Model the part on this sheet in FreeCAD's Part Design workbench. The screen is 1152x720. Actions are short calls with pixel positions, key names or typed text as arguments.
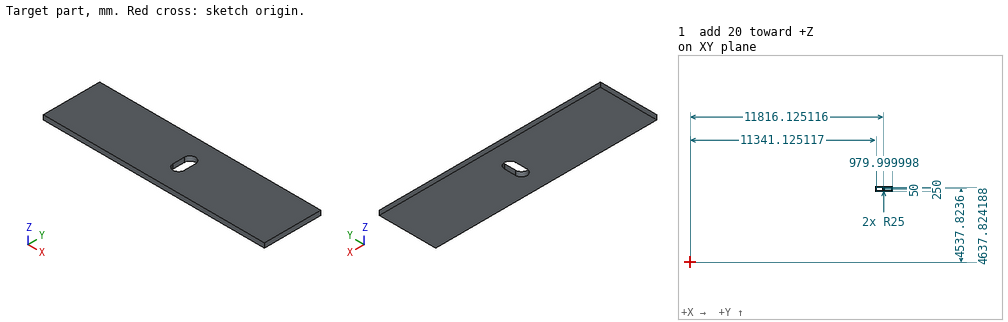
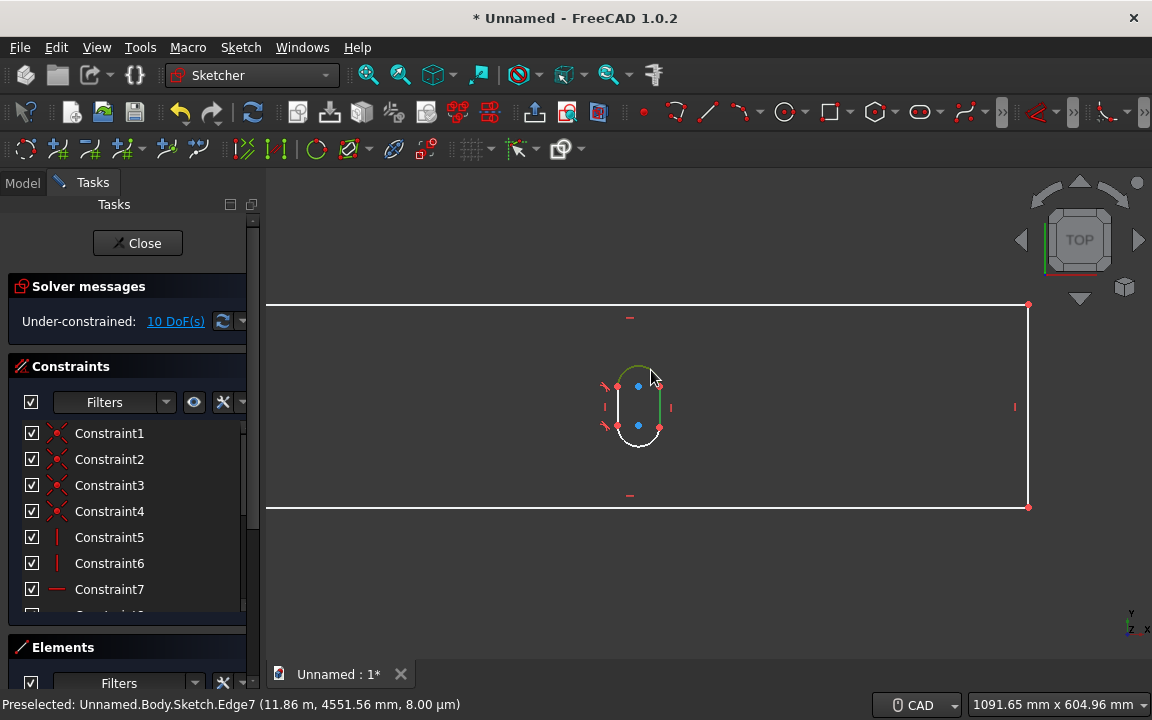
key(t)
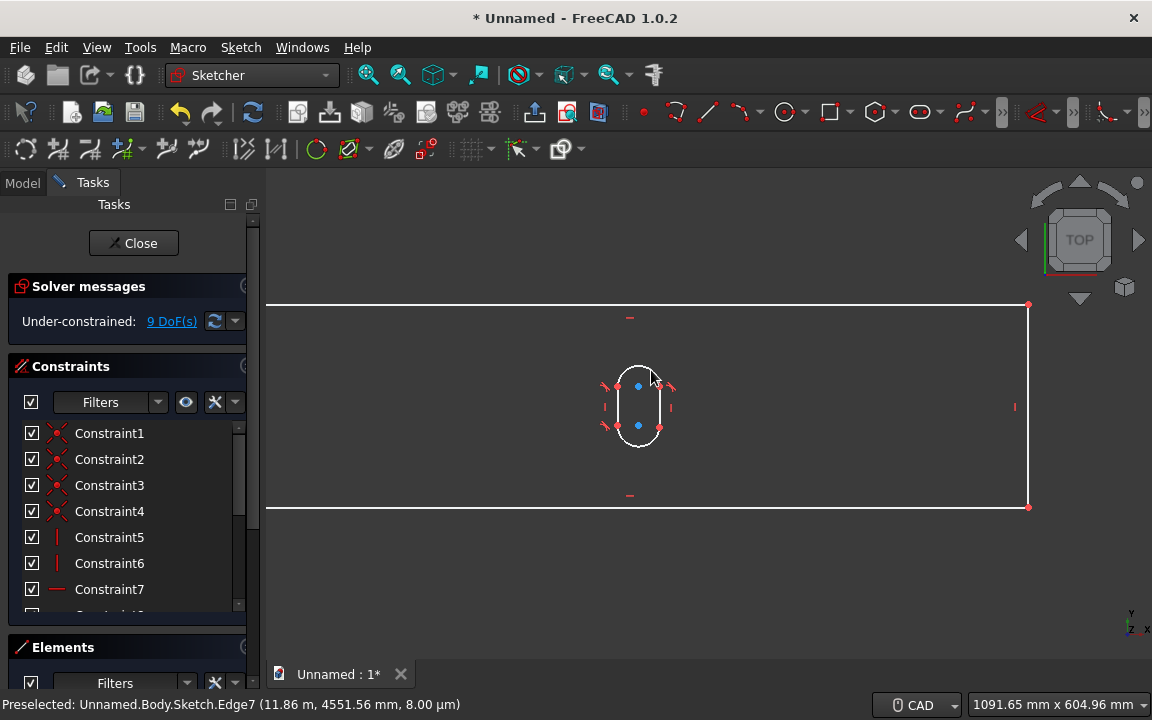
click(660, 399)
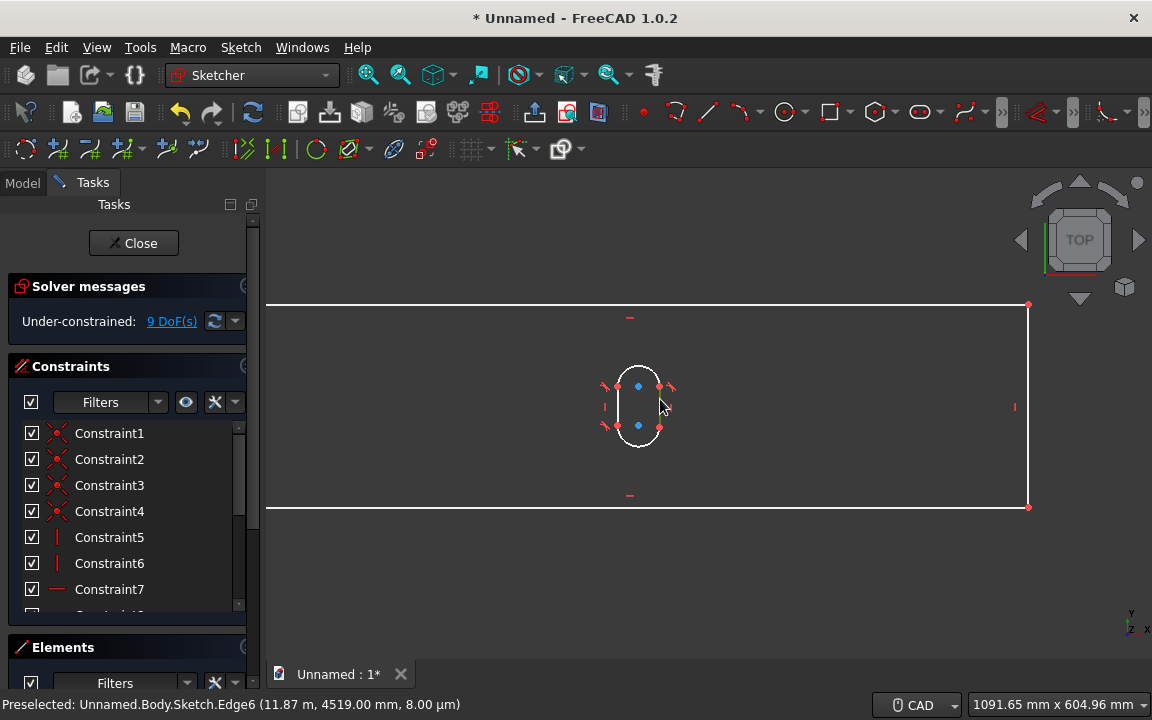
click(626, 442)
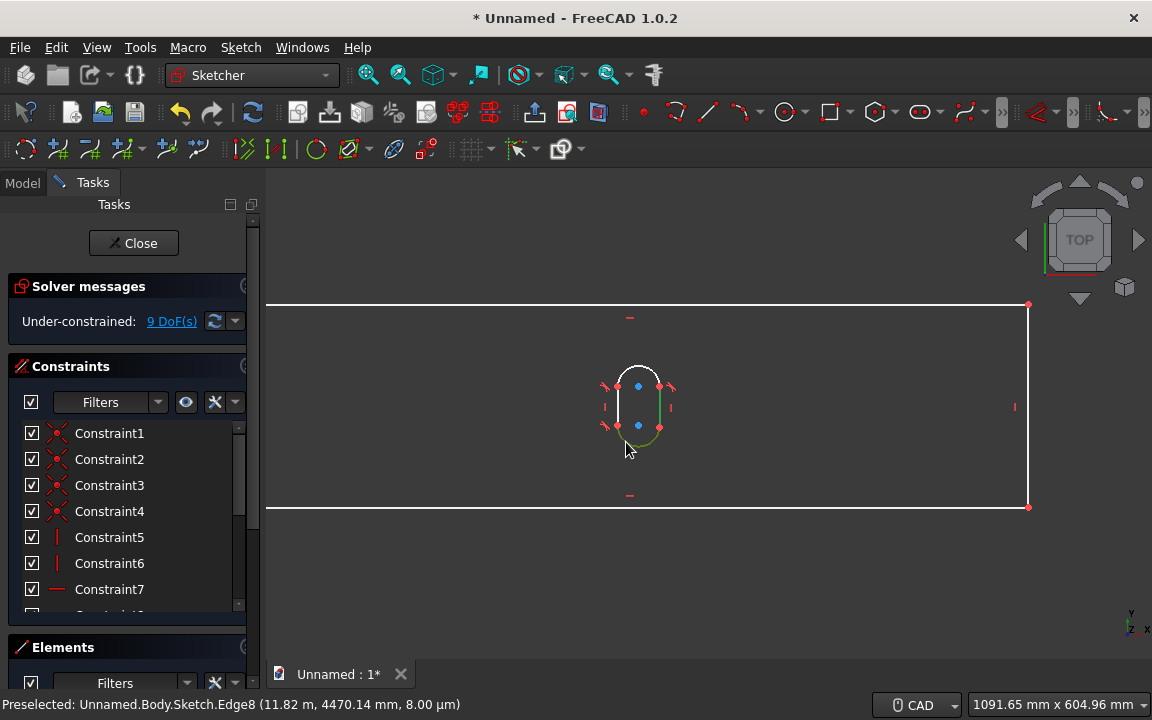
key(t)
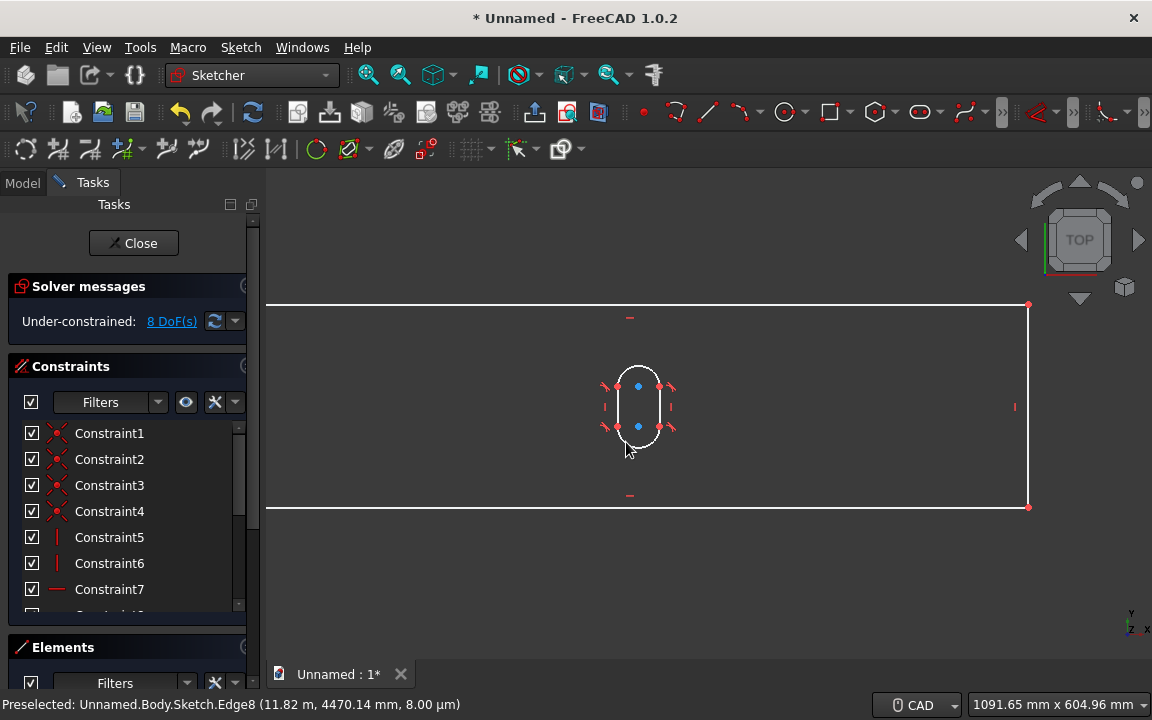
scroll(651, 370, up, 4)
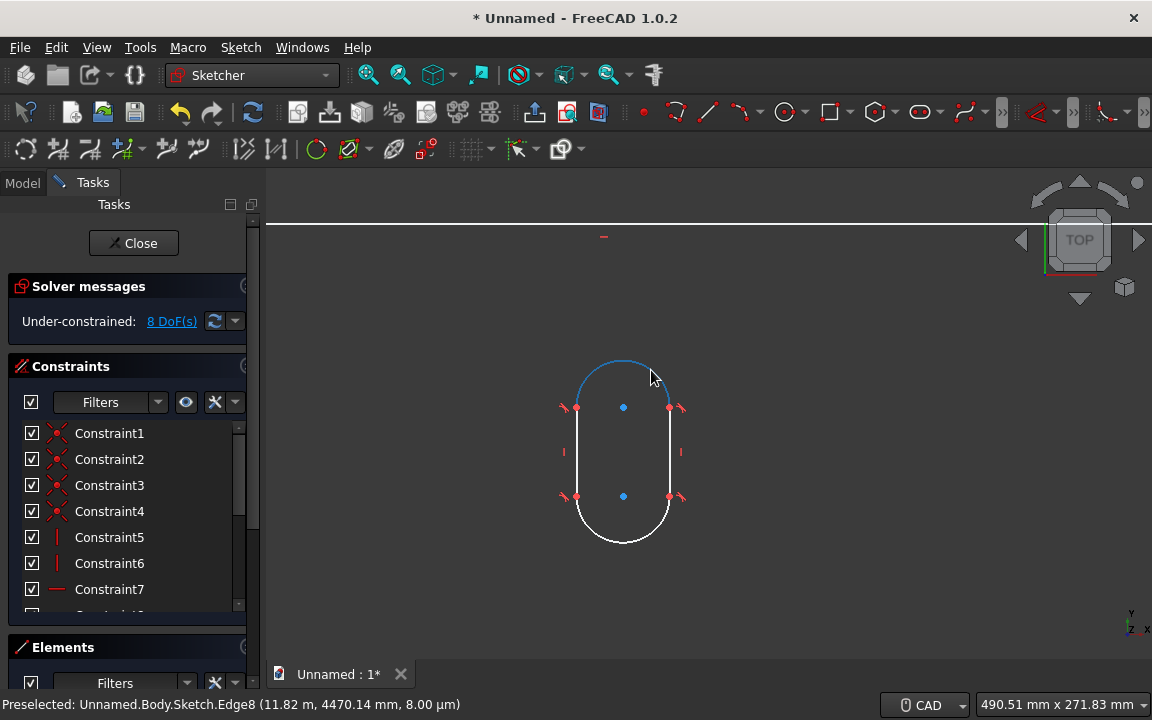
click(650, 369)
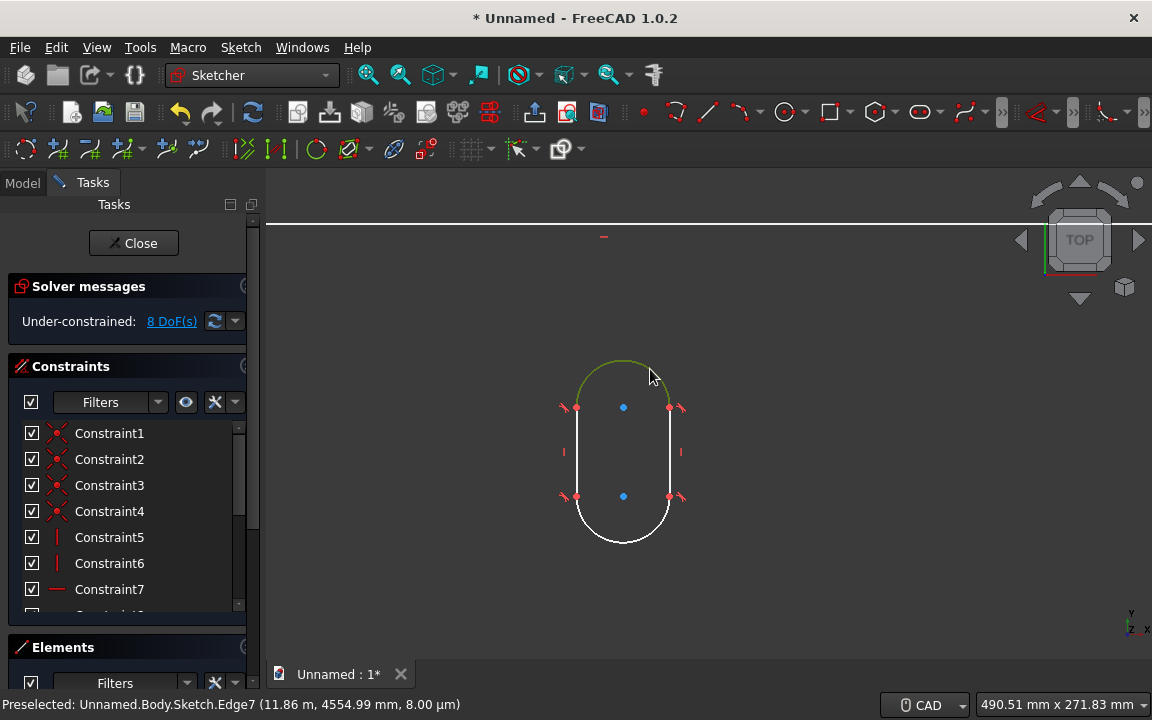
key(k)
key(r)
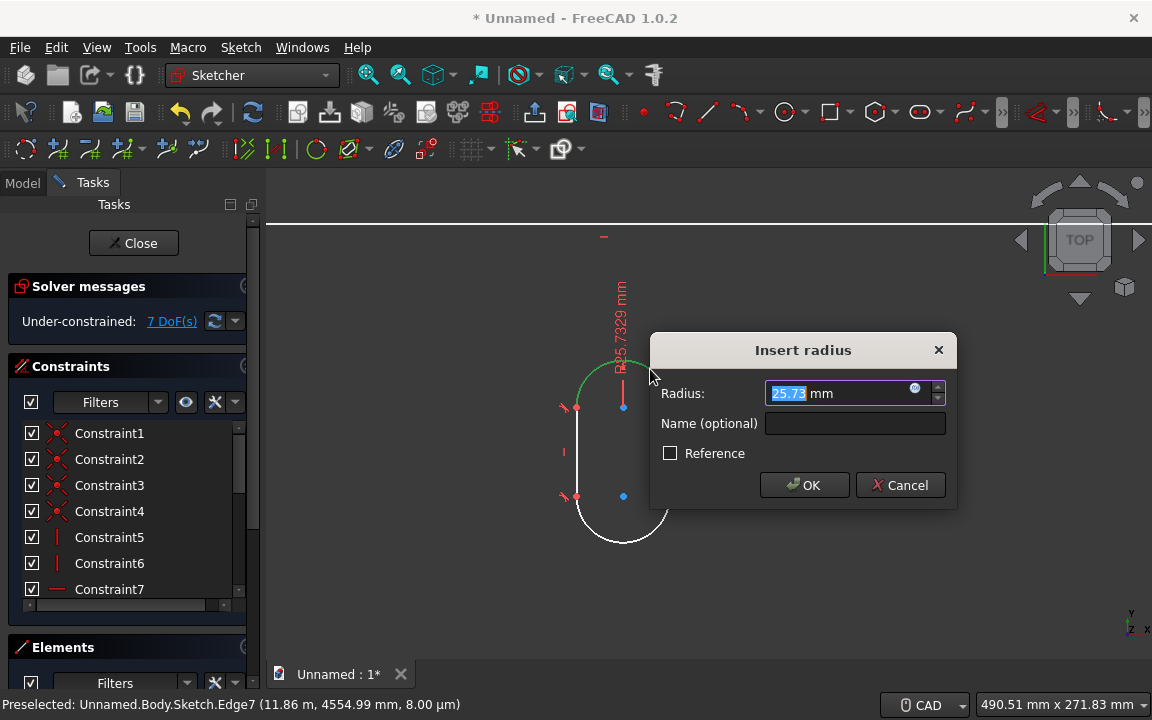
text(25)
key(Return)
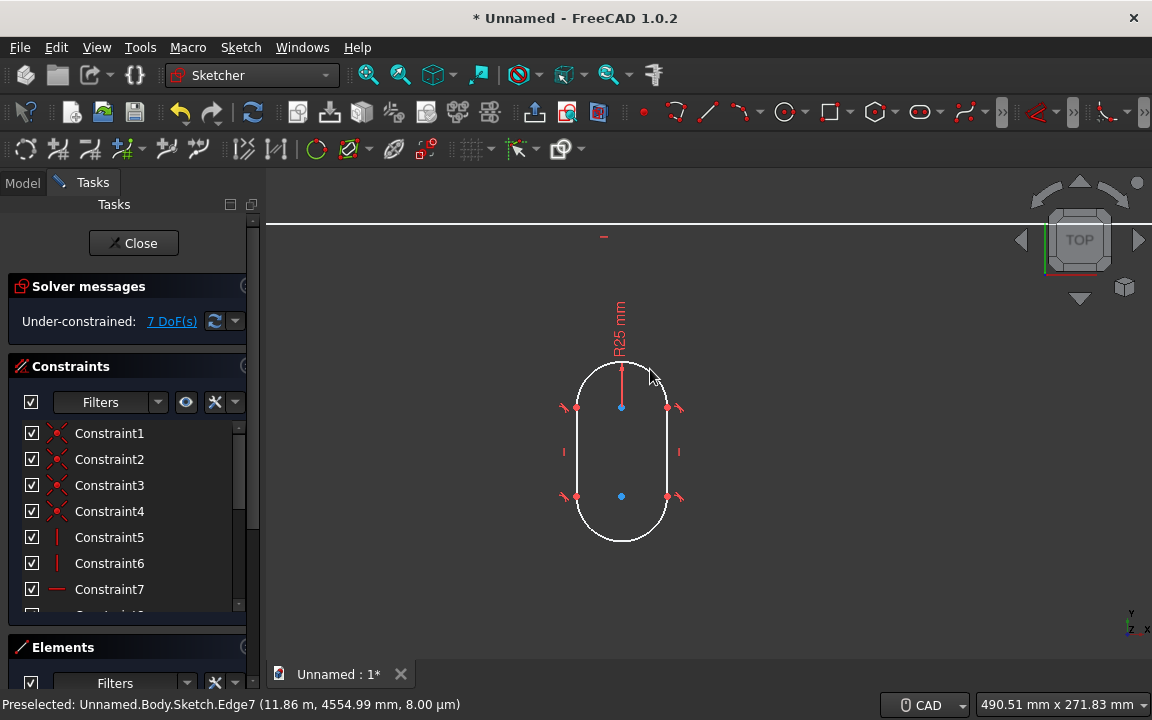
click(577, 469)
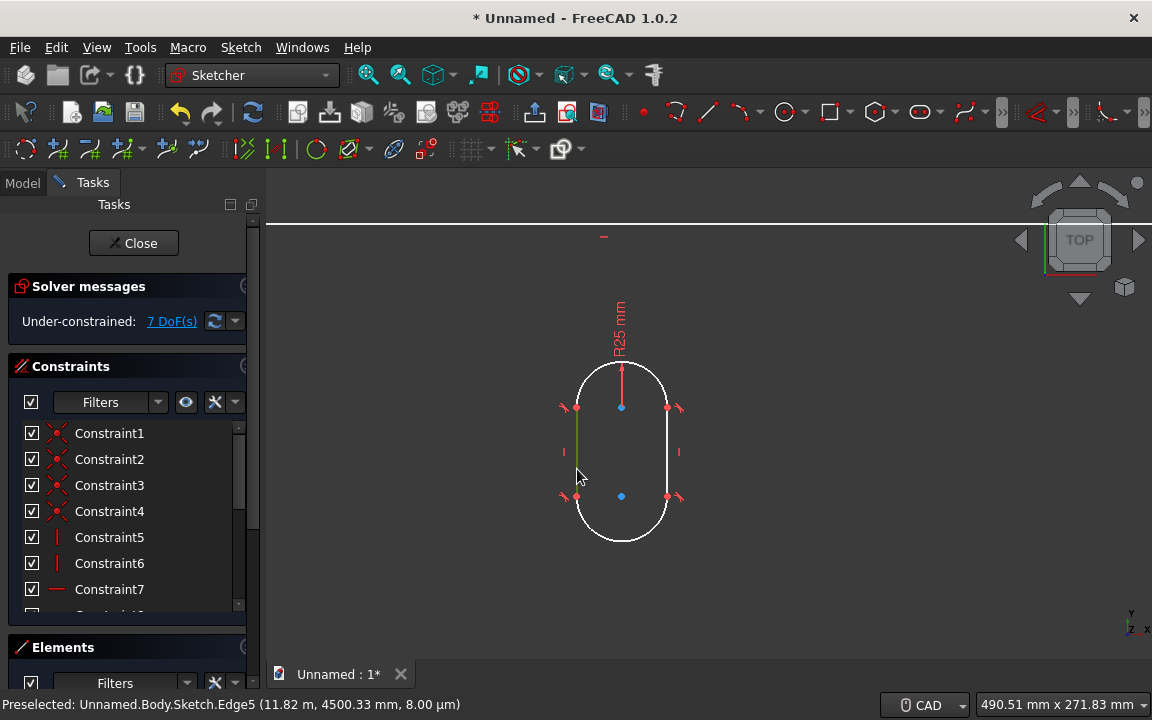
key(i)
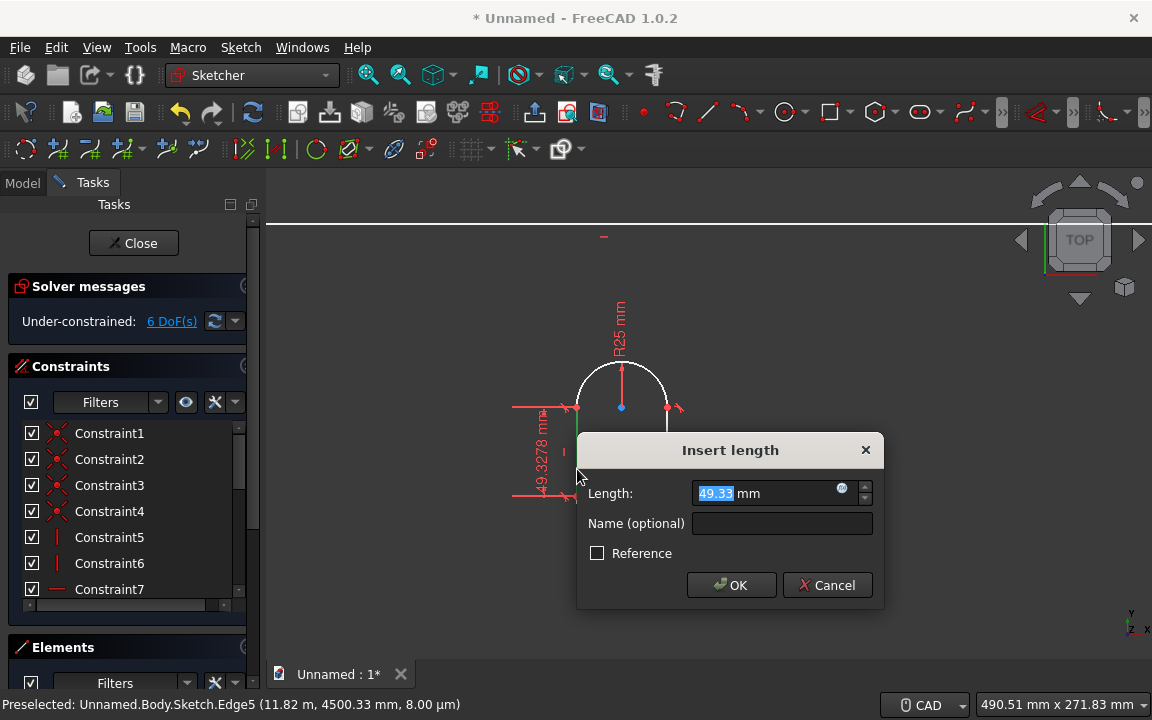
text(50)
key(Return)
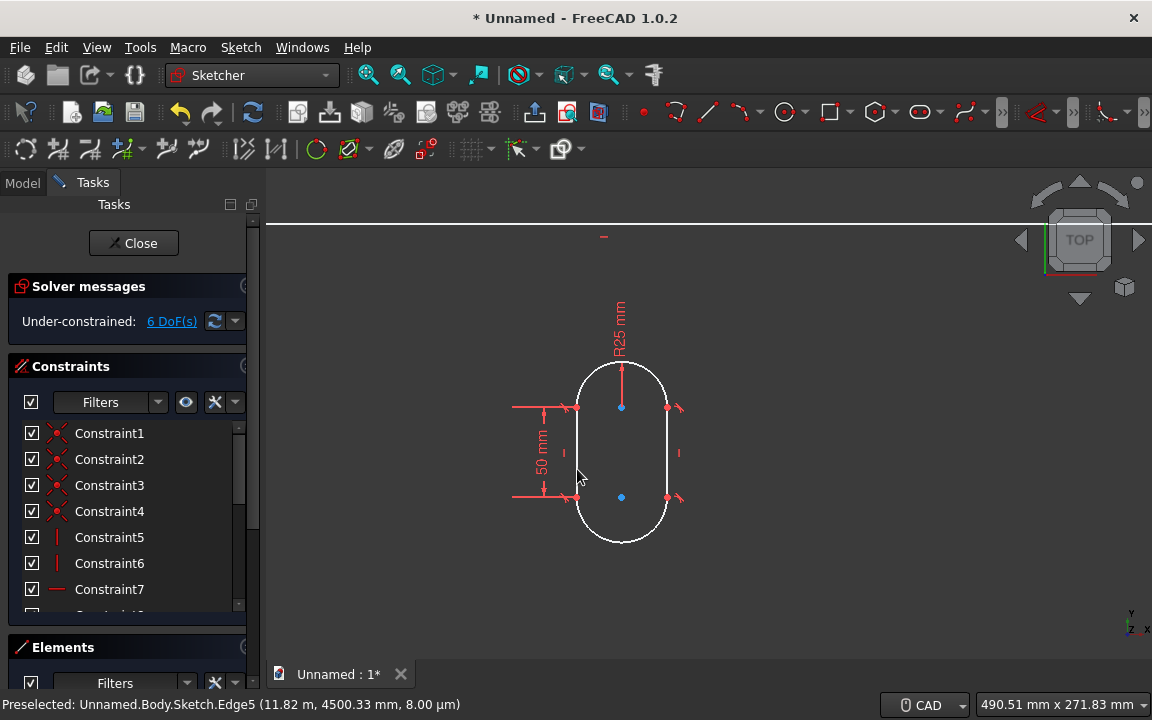
scroll(656, 399, down, 6)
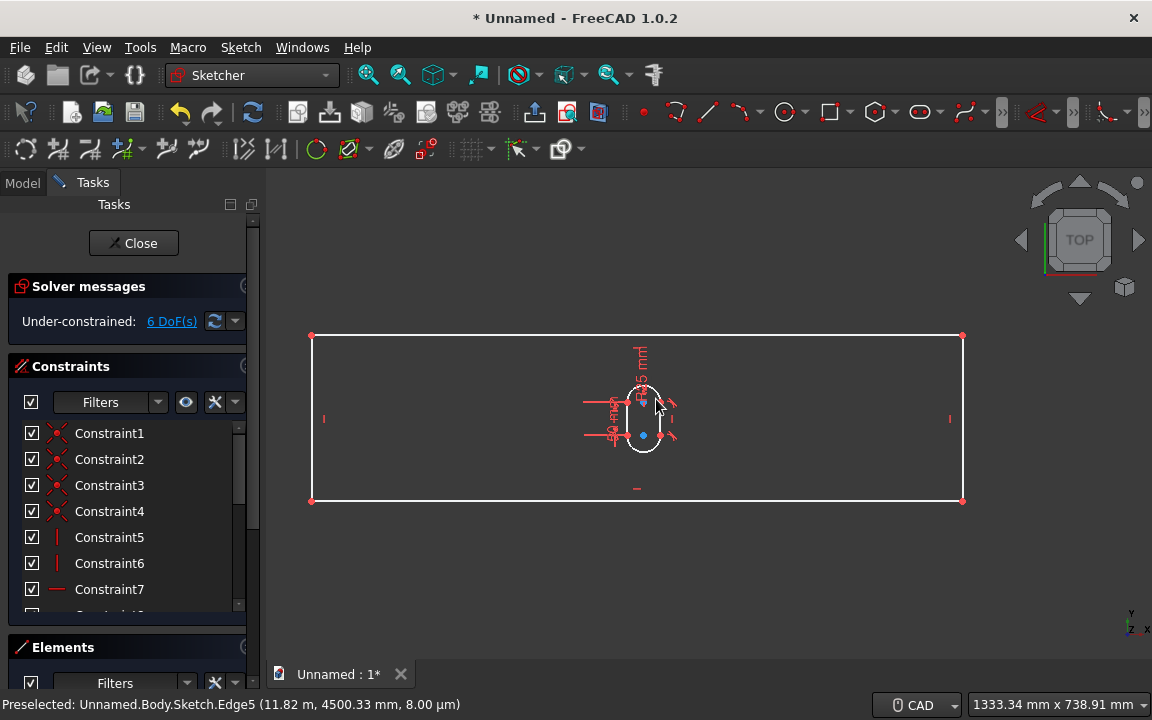
click(374, 388)